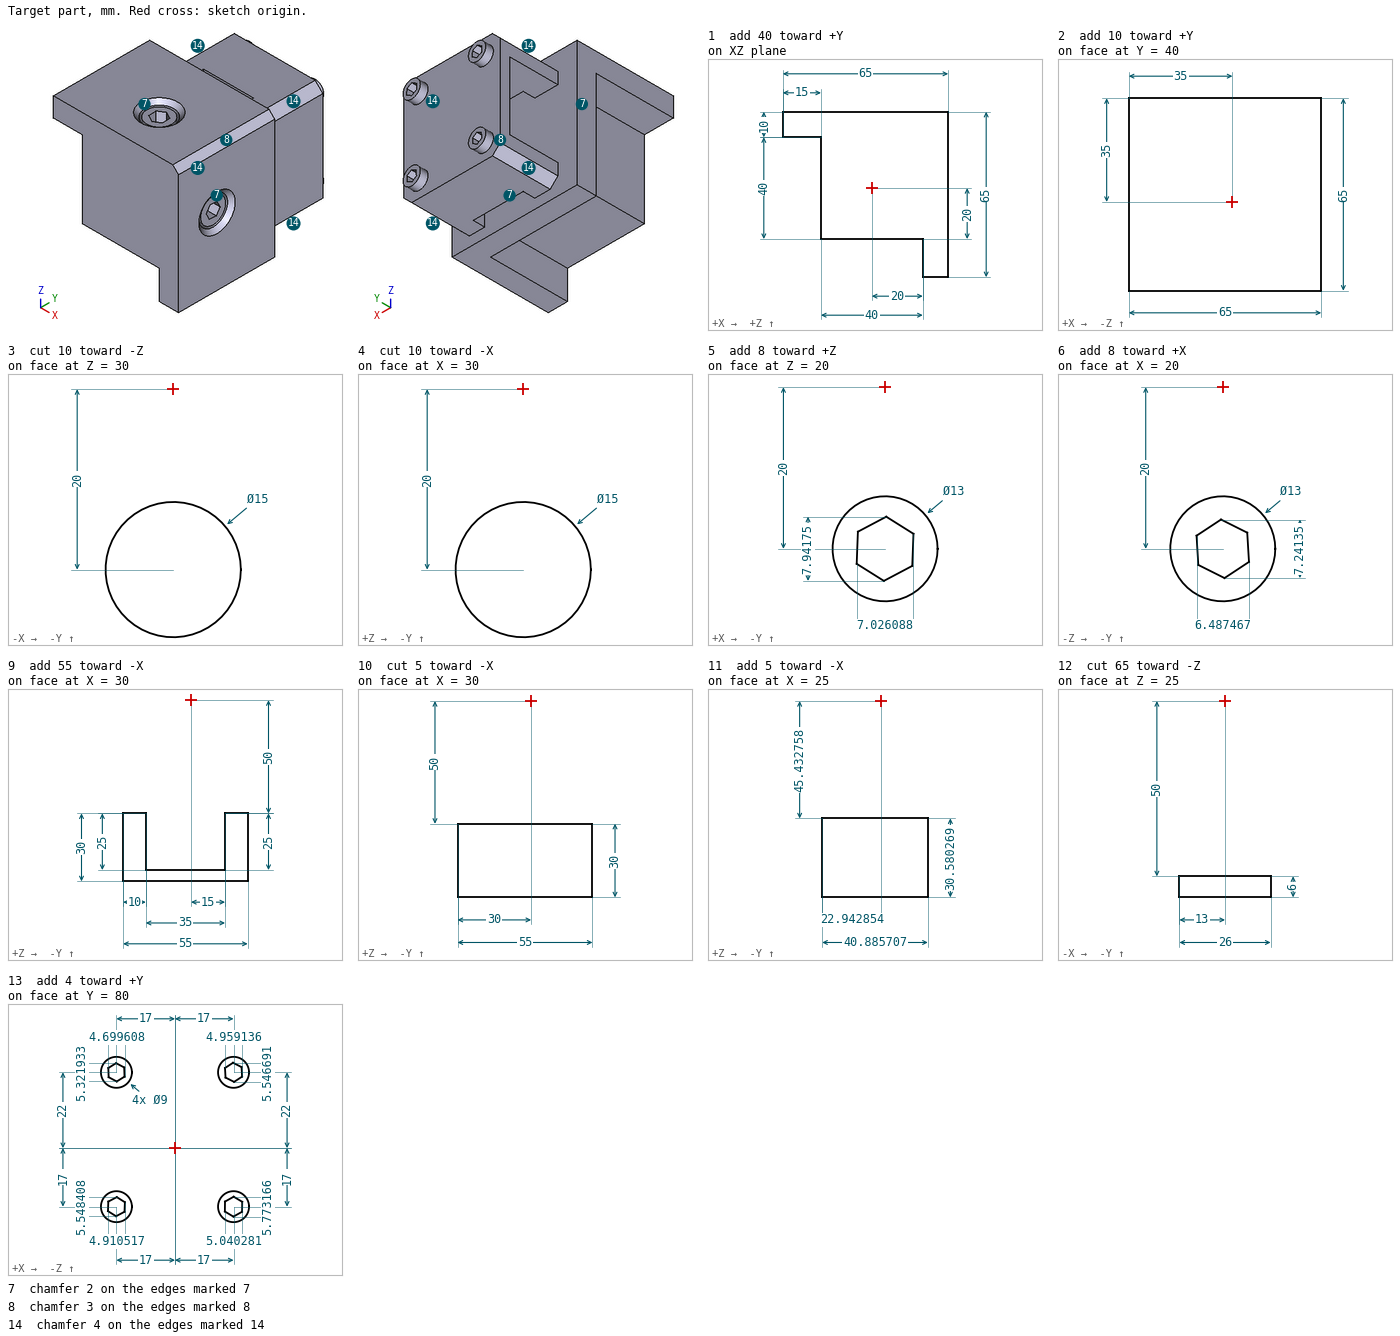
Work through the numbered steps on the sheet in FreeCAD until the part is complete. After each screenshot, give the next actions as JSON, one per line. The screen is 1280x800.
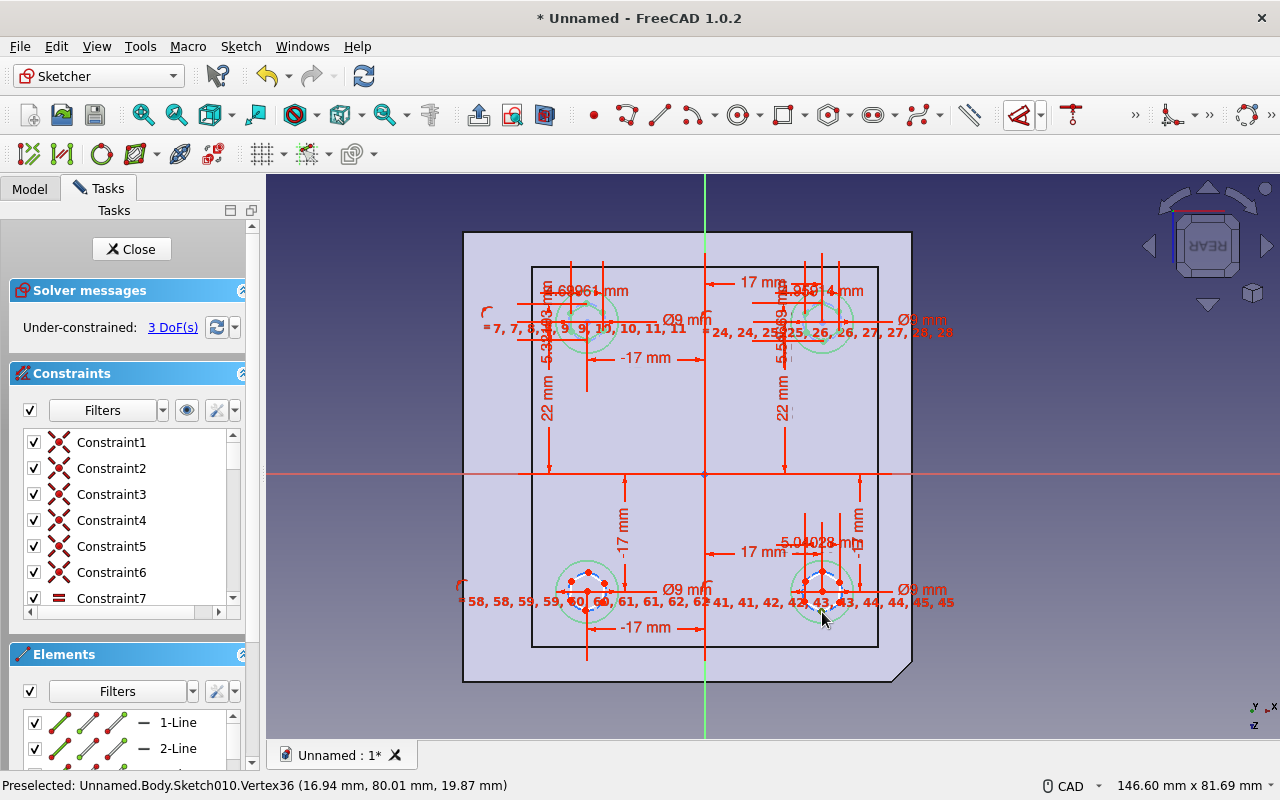
{"action": "left_click", "coordinate": [823, 572]}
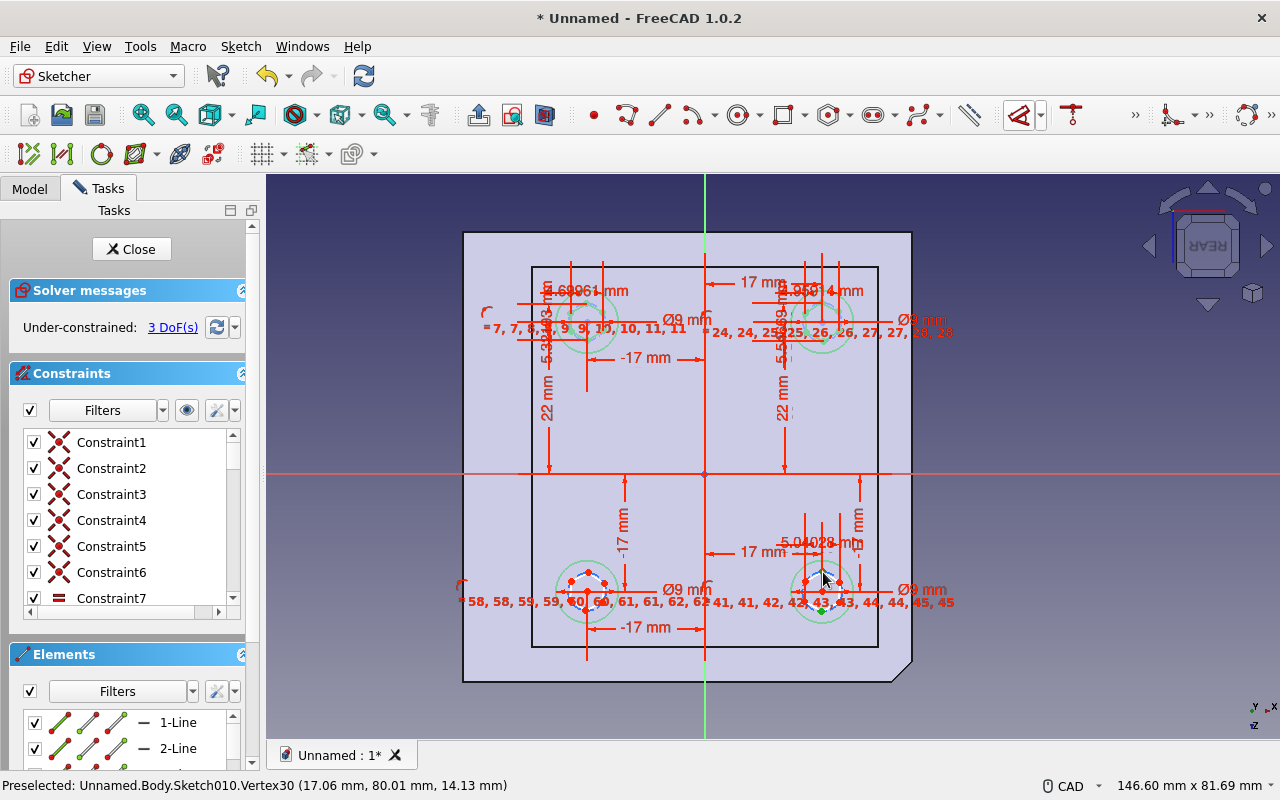
{"action": "key", "text": "i"}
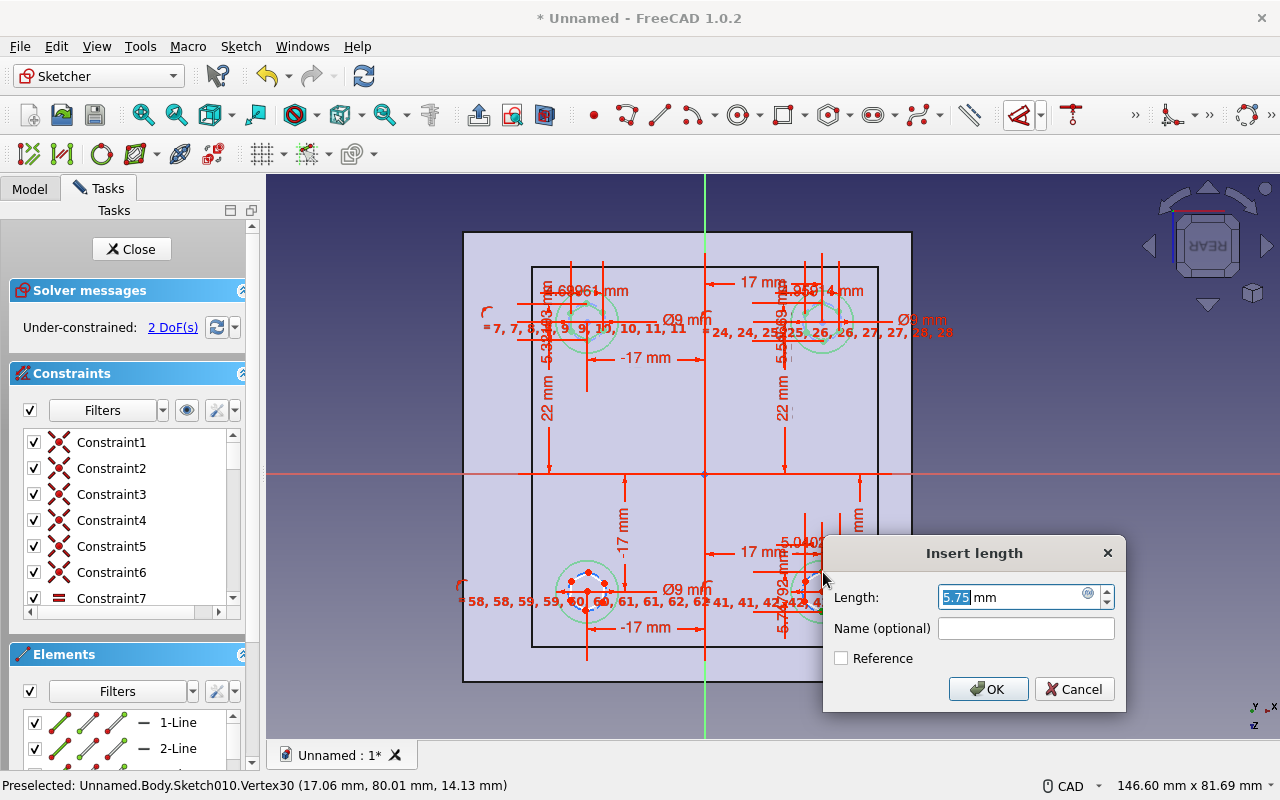
{"action": "type", "text": "5.773166"}
{"action": "key", "text": "Return"}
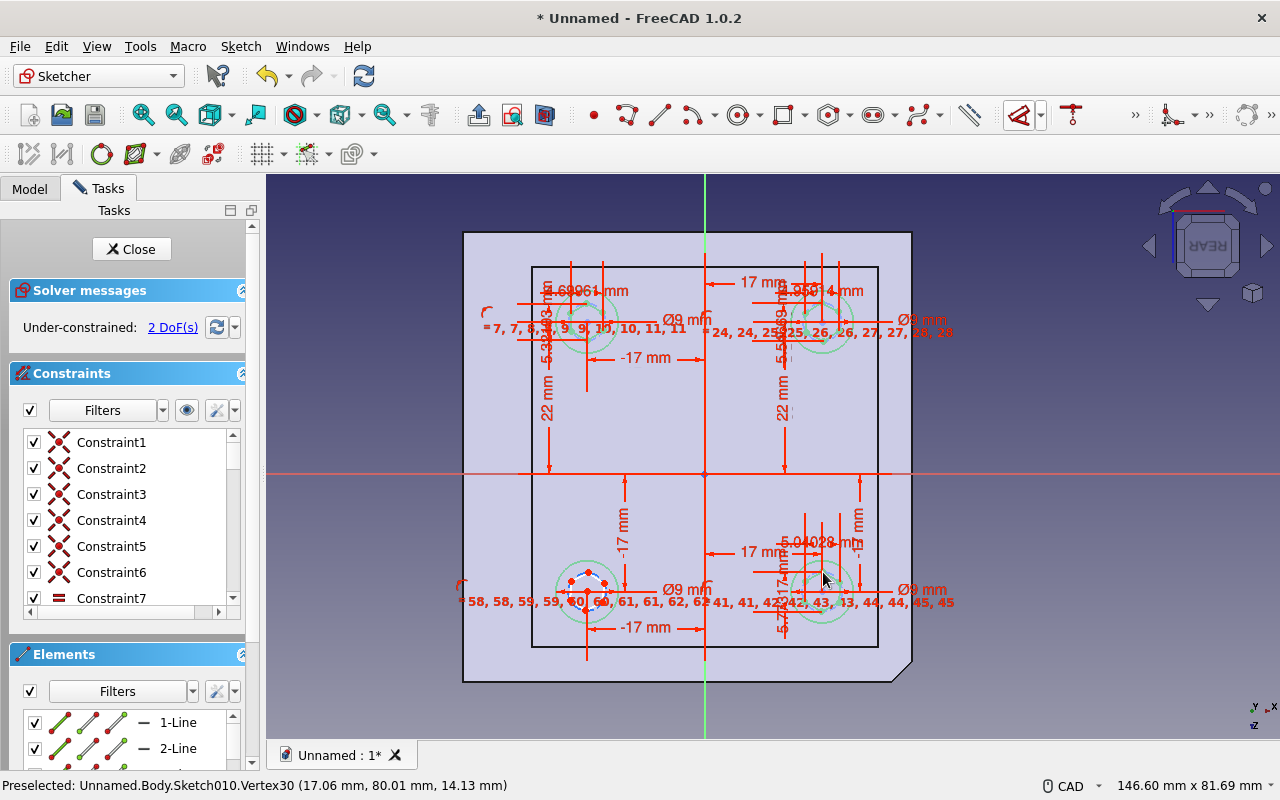
{"action": "left_click", "coordinate": [570, 600]}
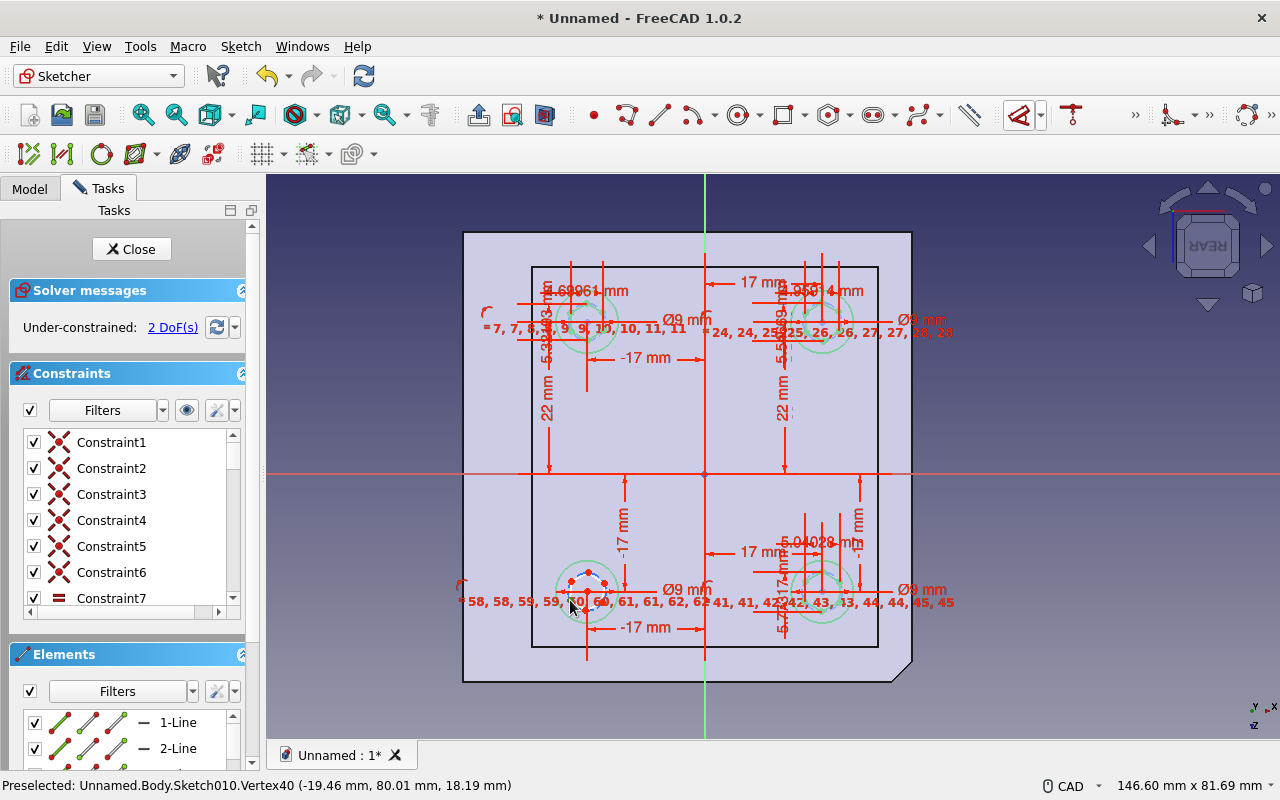
{"action": "left_click", "coordinate": [604, 584]}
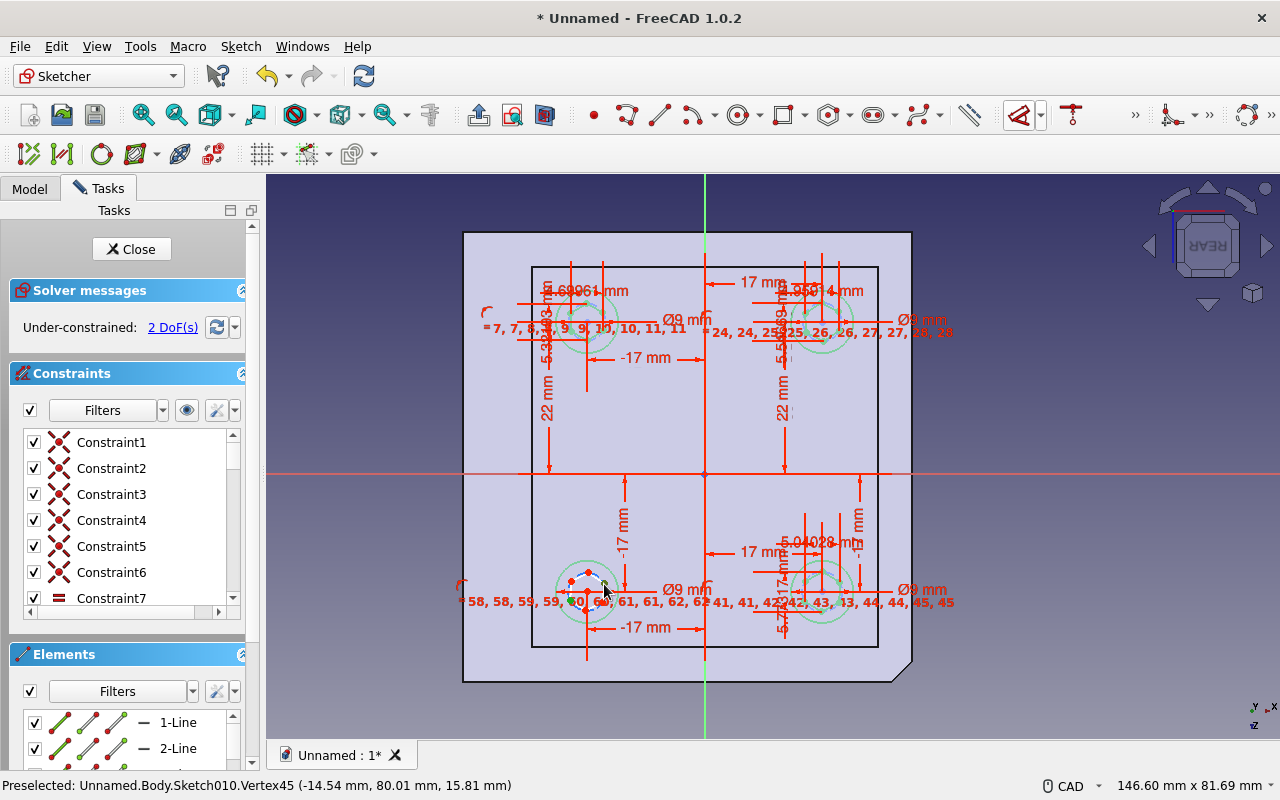
{"action": "key", "text": "l"}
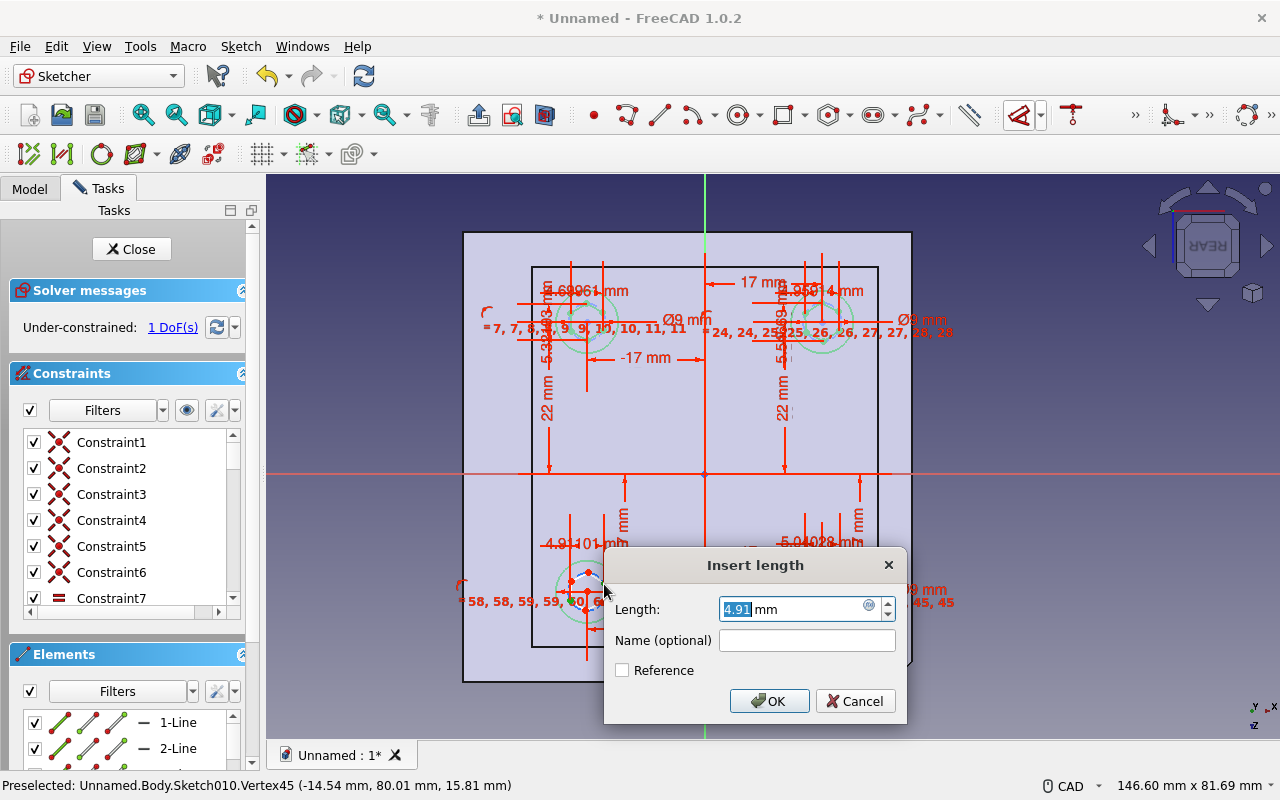
{"action": "type", "text": "4.910517"}
{"action": "key", "text": "Return"}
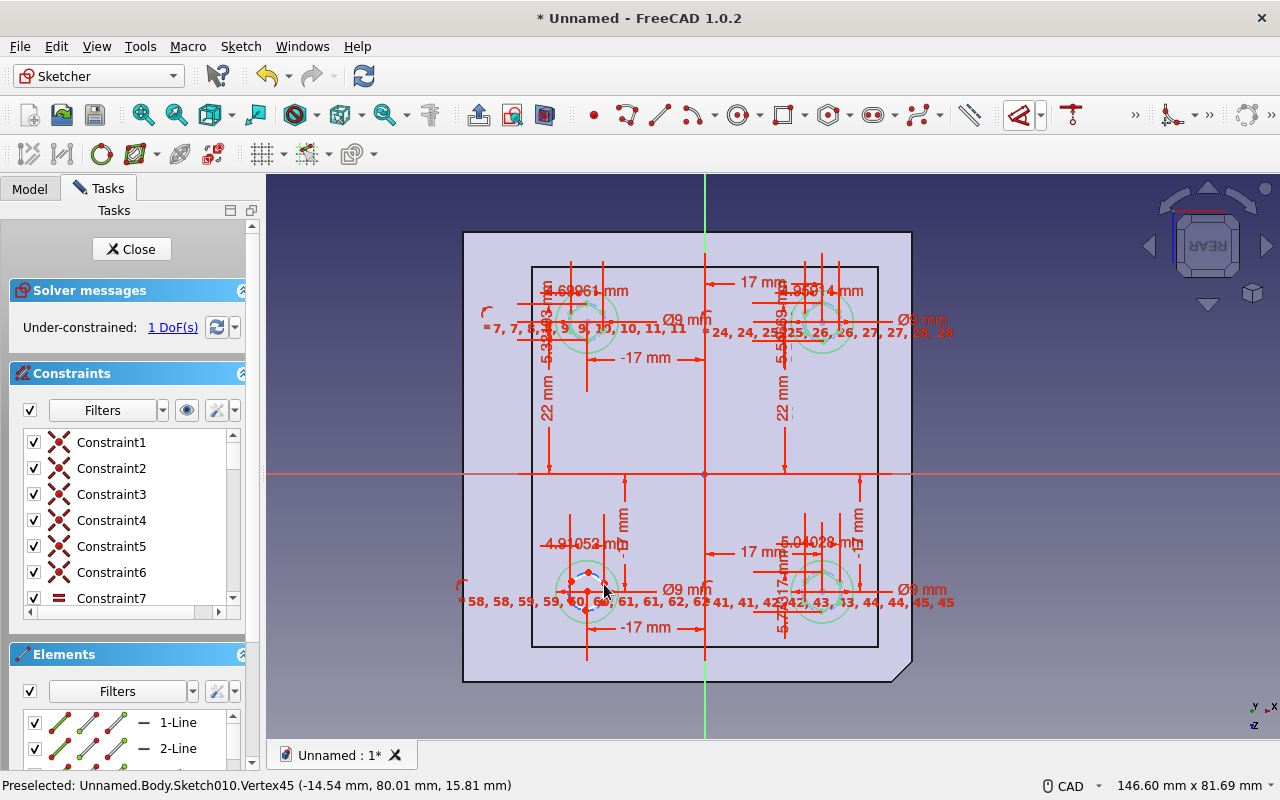
{"action": "left_click", "coordinate": [586, 611]}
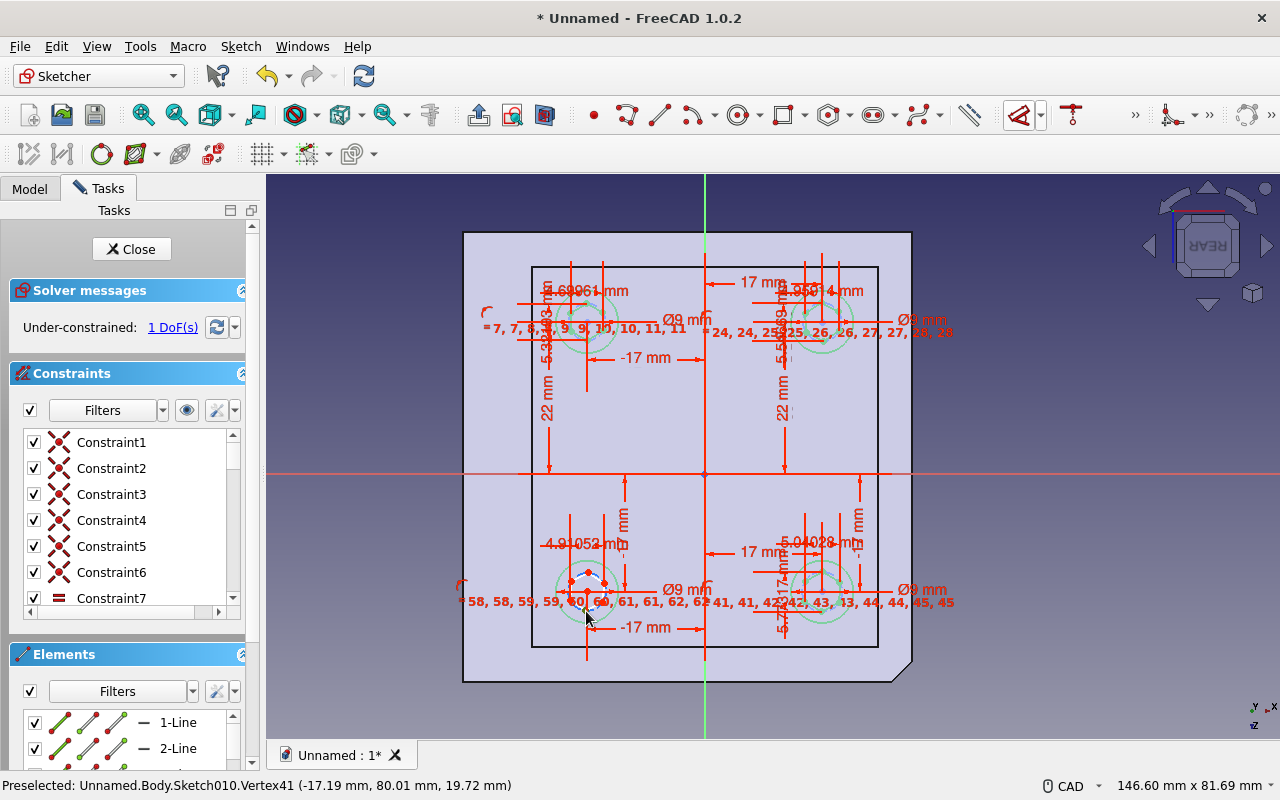
{"action": "left_click", "coordinate": [588, 573]}